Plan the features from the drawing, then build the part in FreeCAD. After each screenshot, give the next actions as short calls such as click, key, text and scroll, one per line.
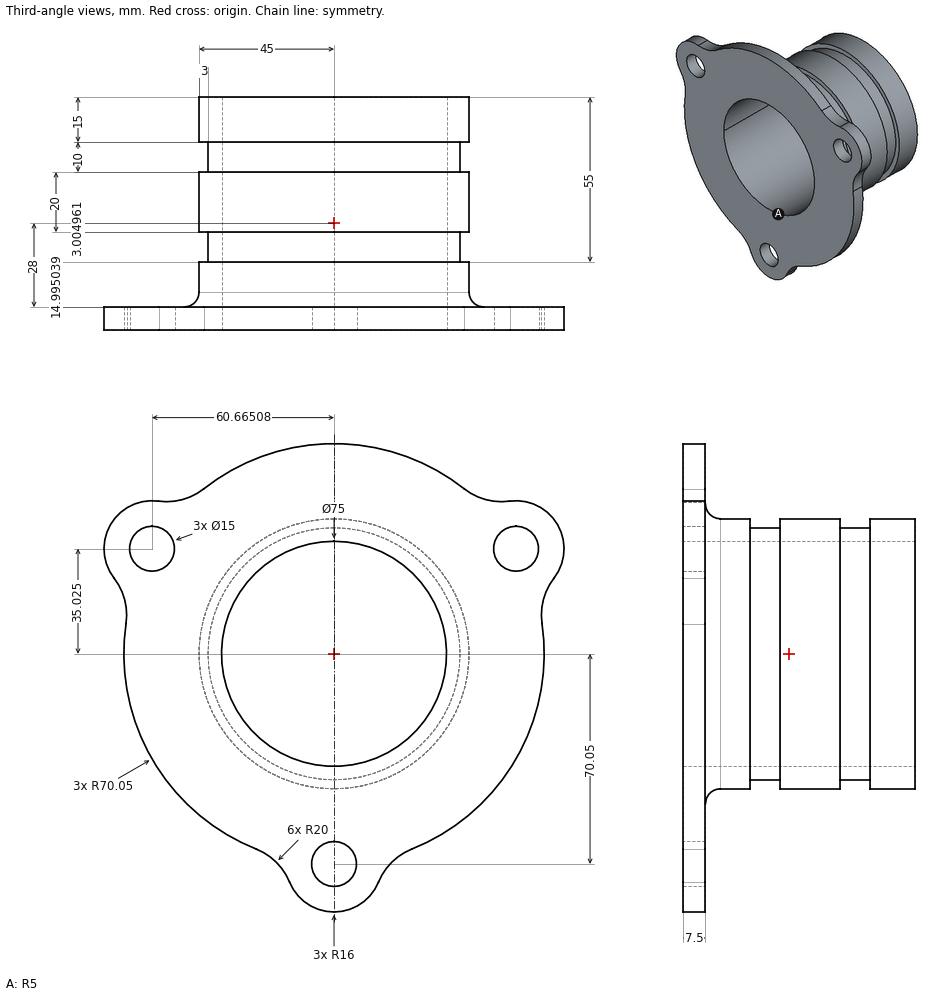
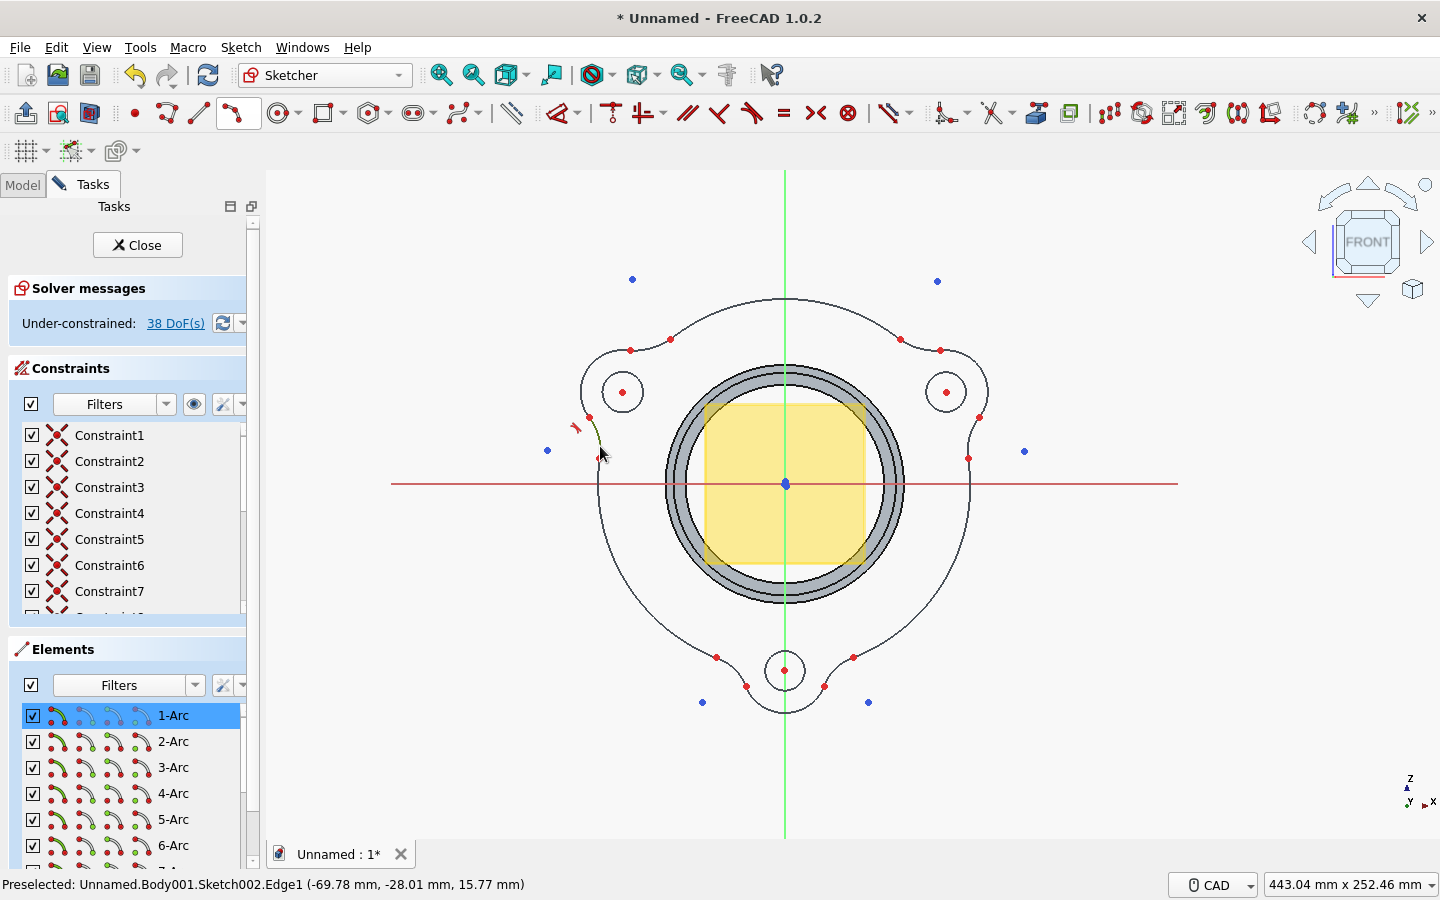
click(605, 533)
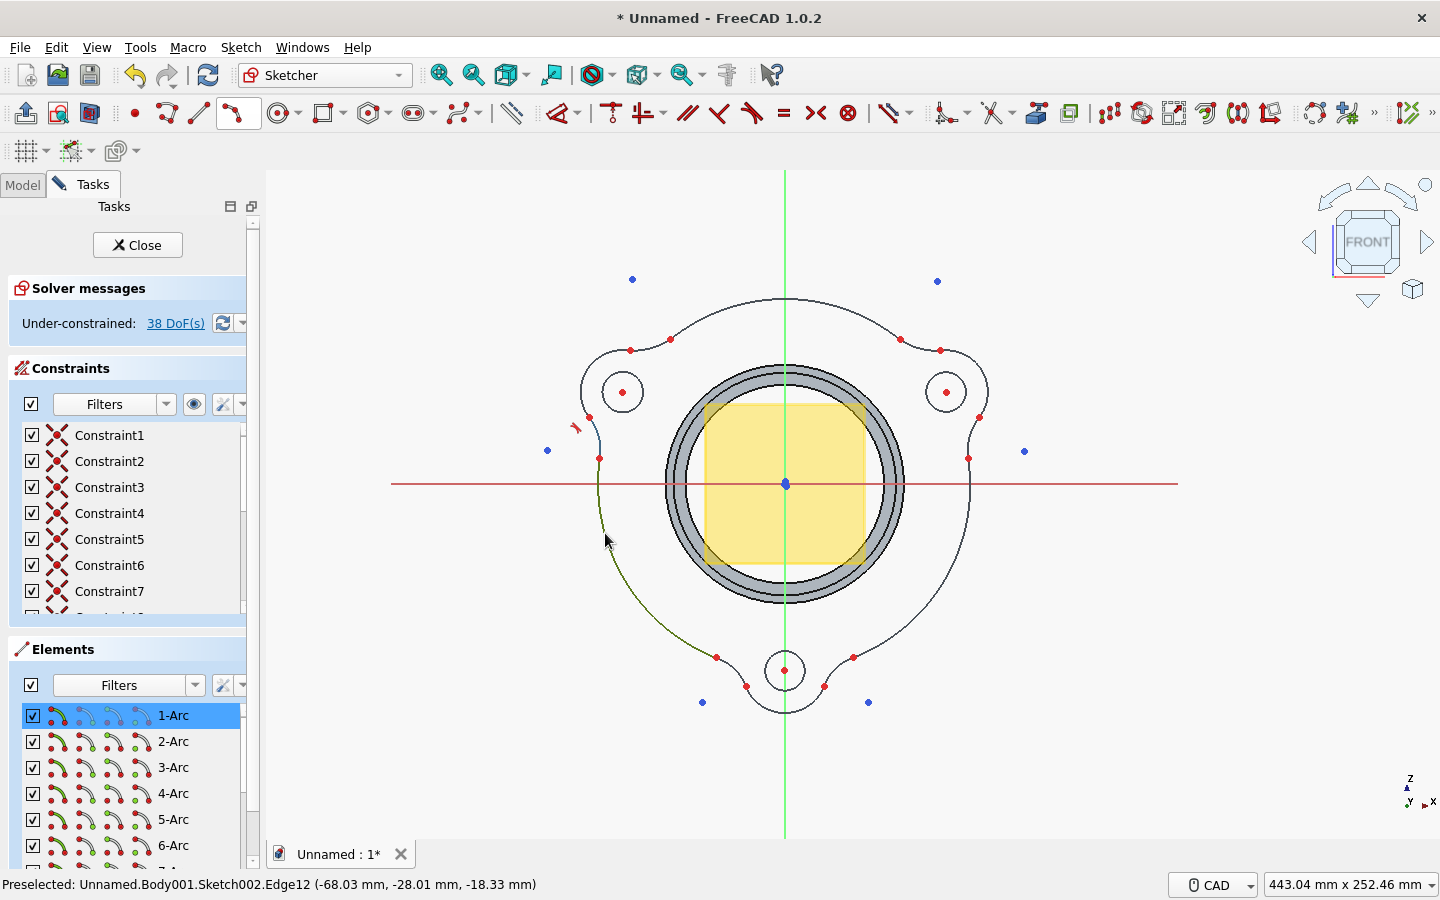
click(752, 114)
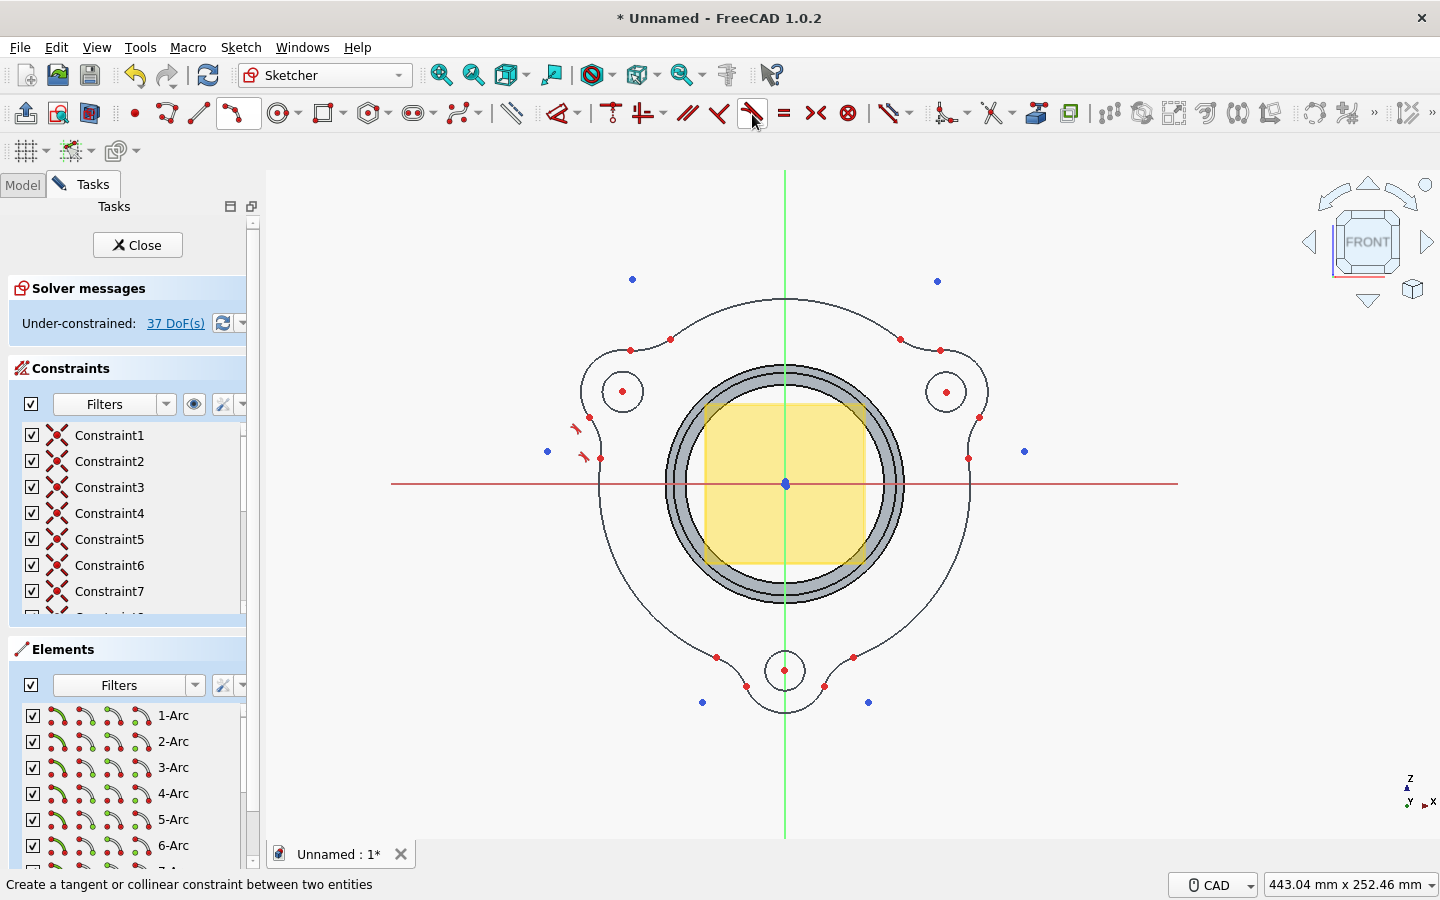
click(601, 356)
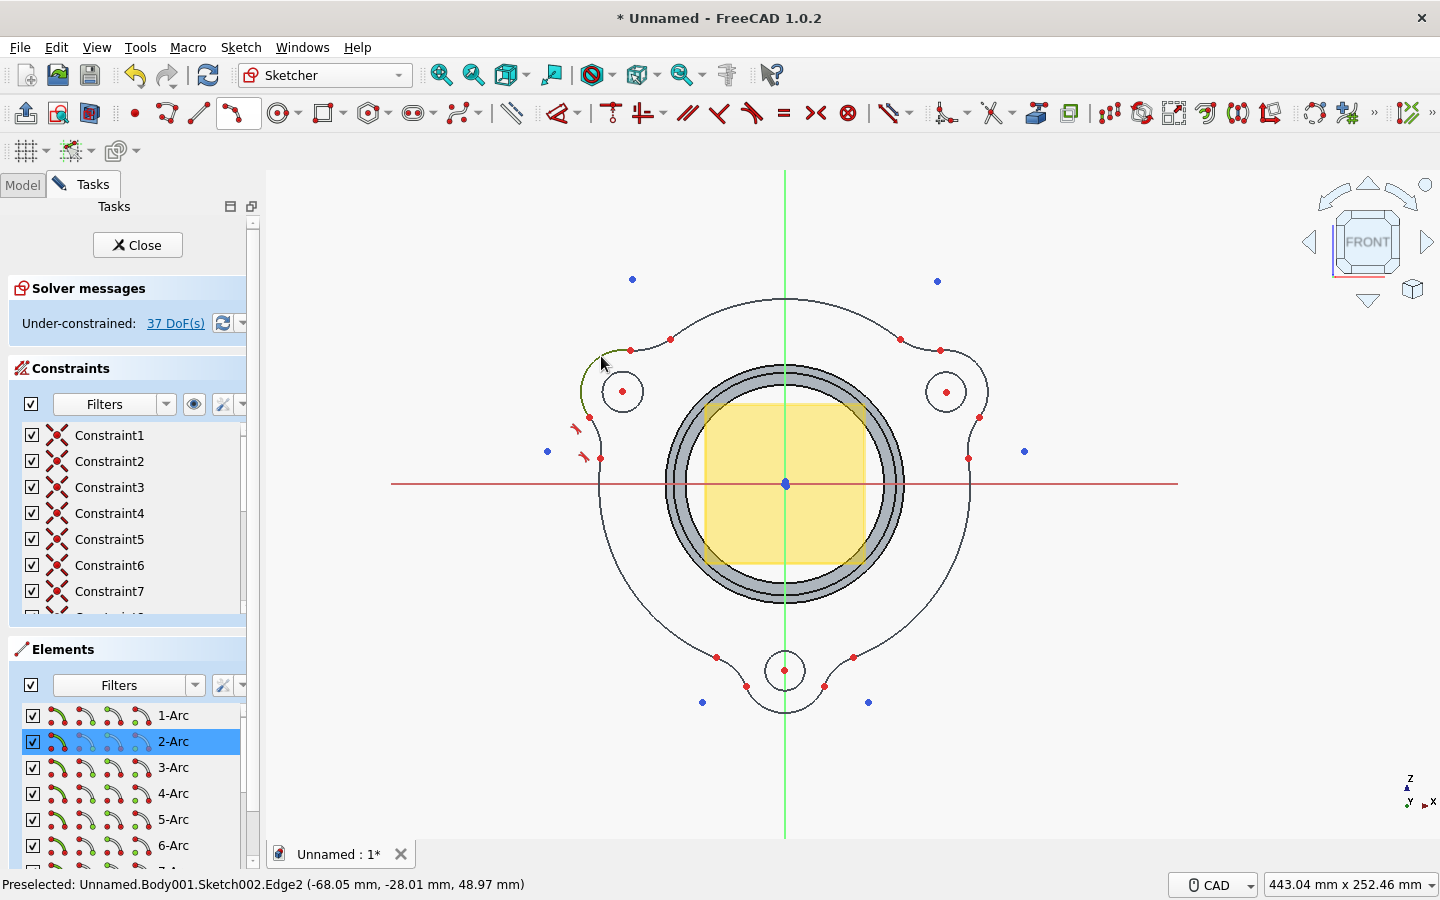
click(643, 350)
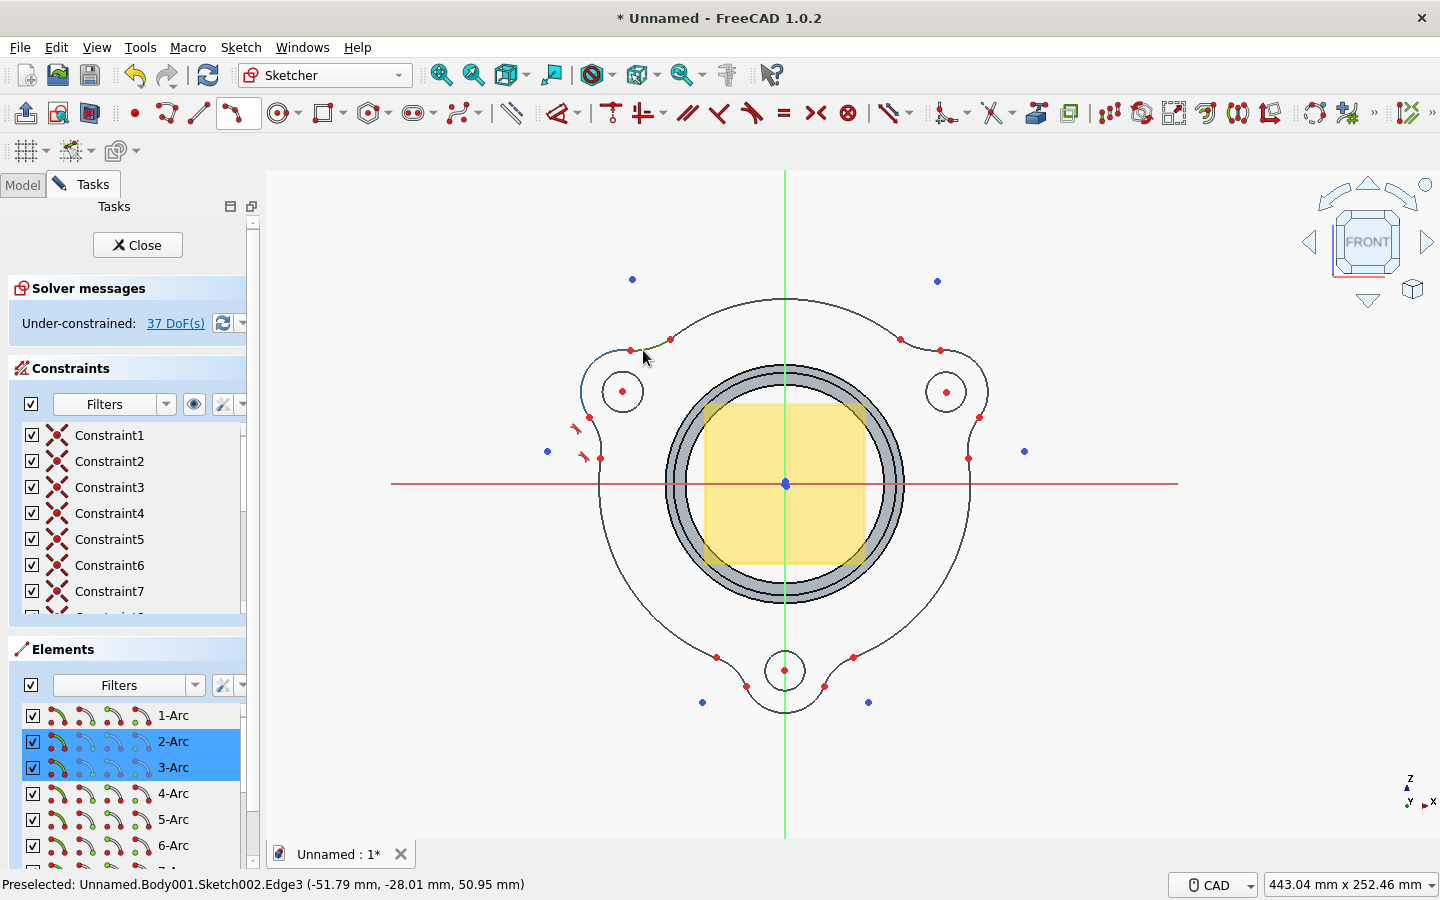
key(t)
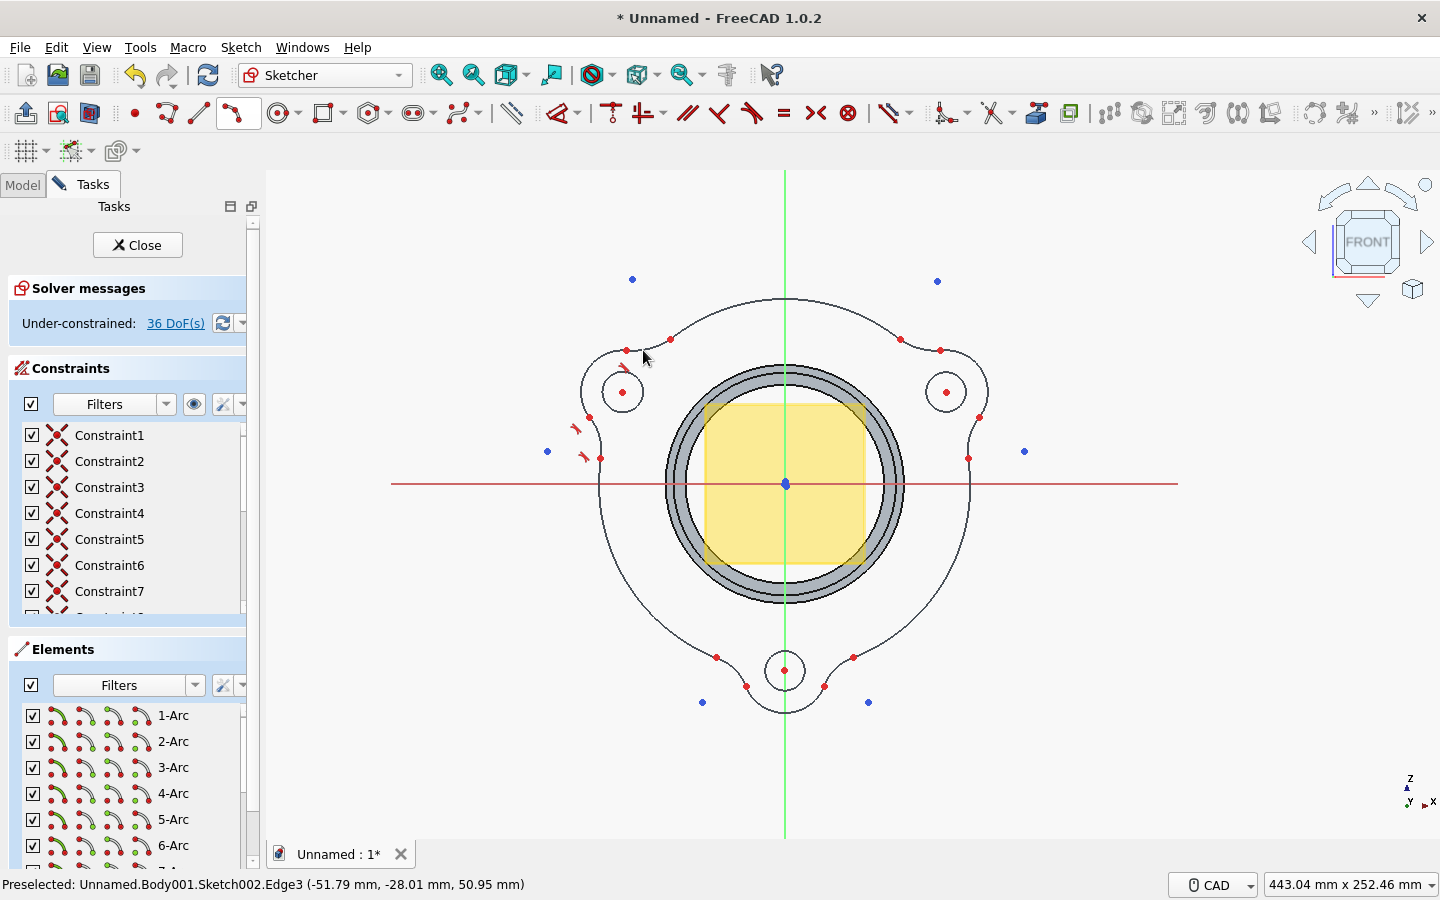
click(640, 350)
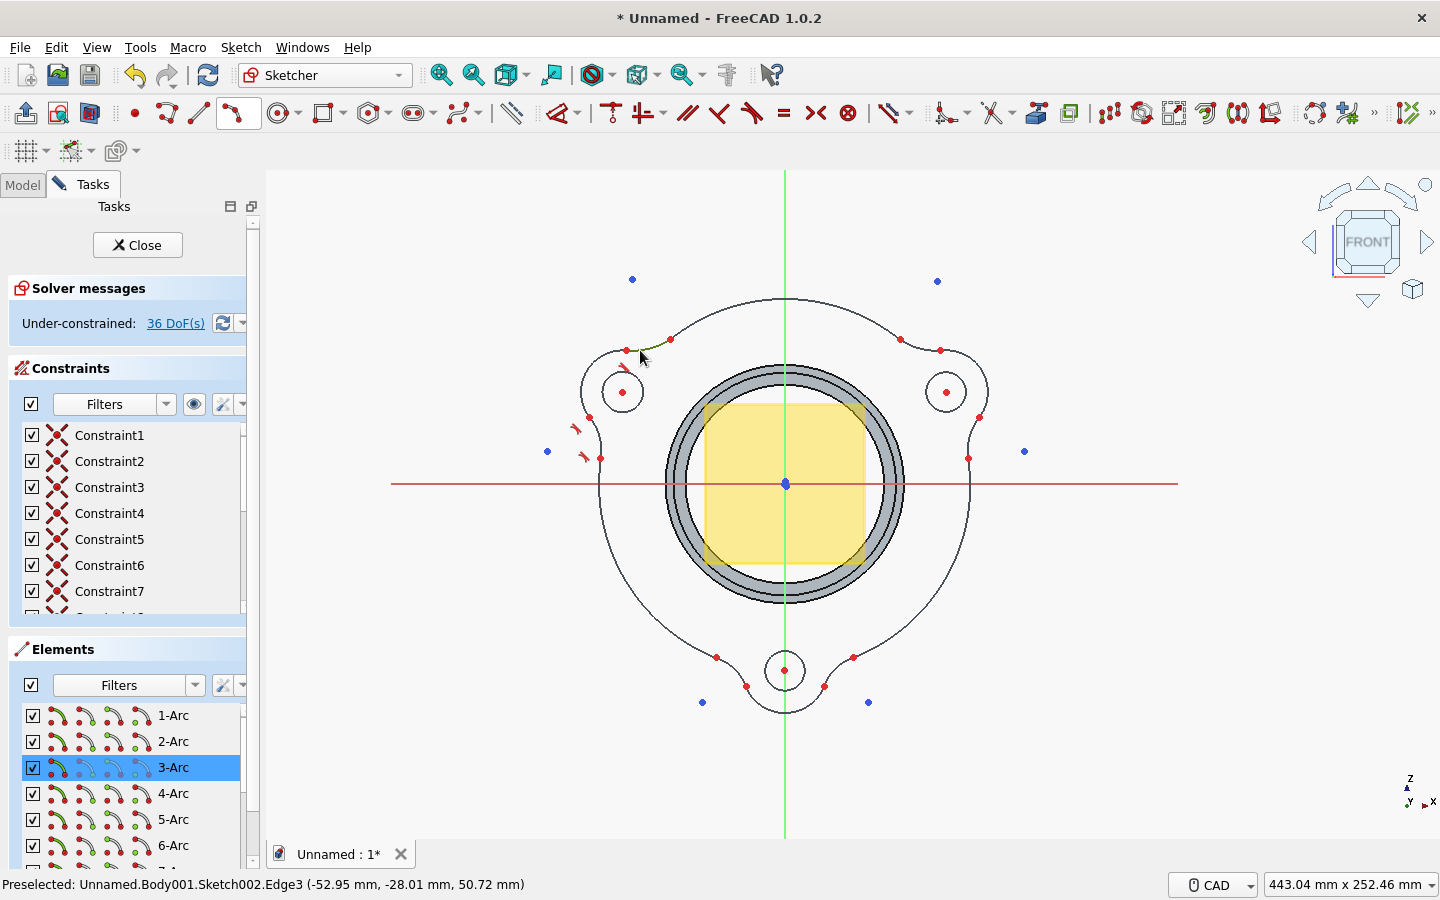
click(834, 306)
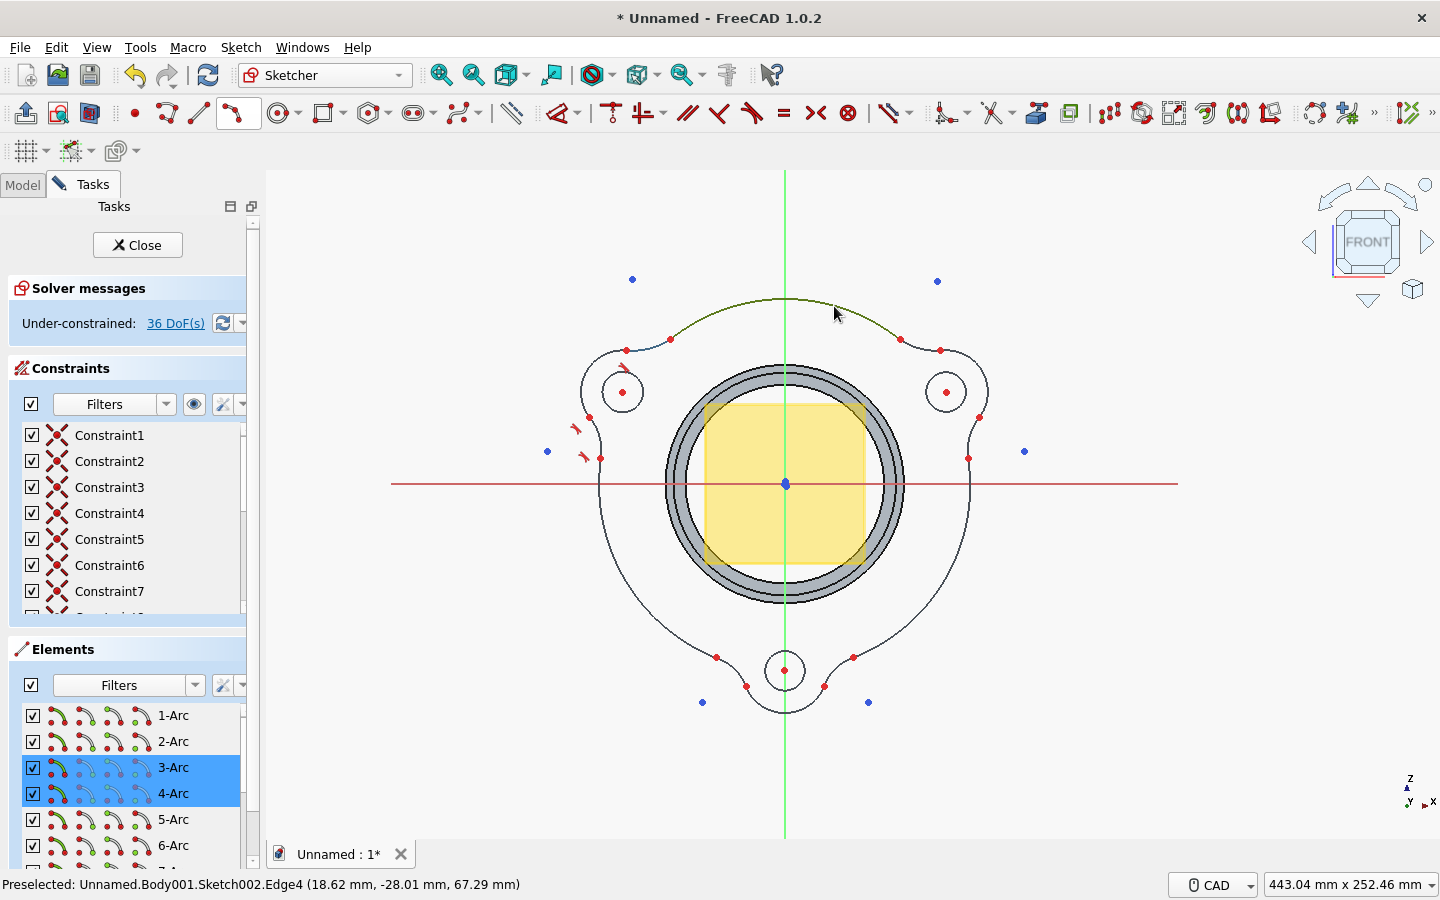
key(t)